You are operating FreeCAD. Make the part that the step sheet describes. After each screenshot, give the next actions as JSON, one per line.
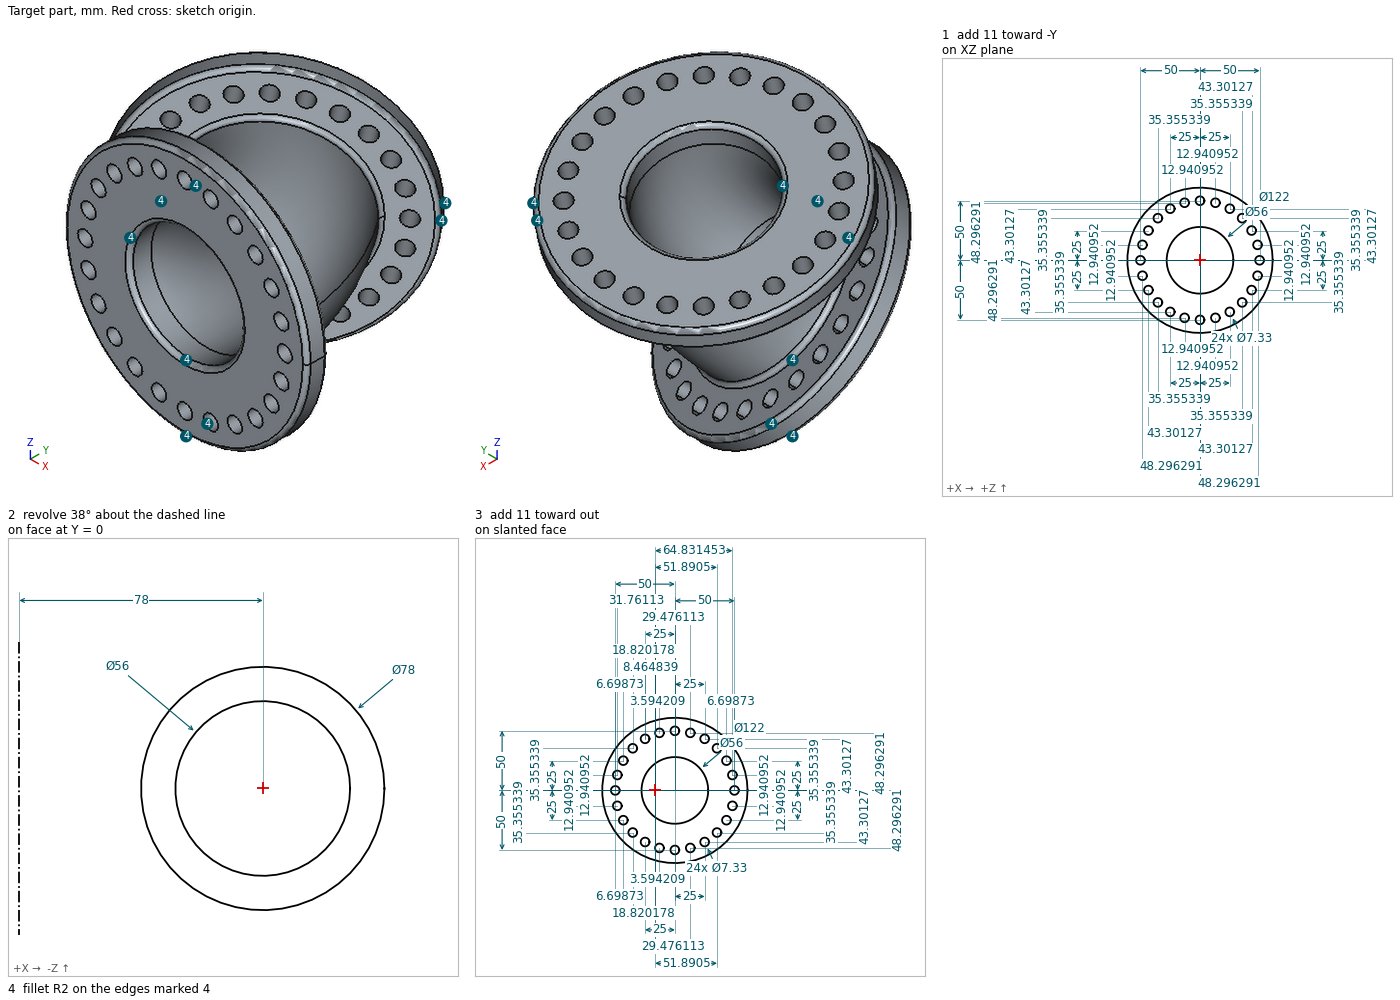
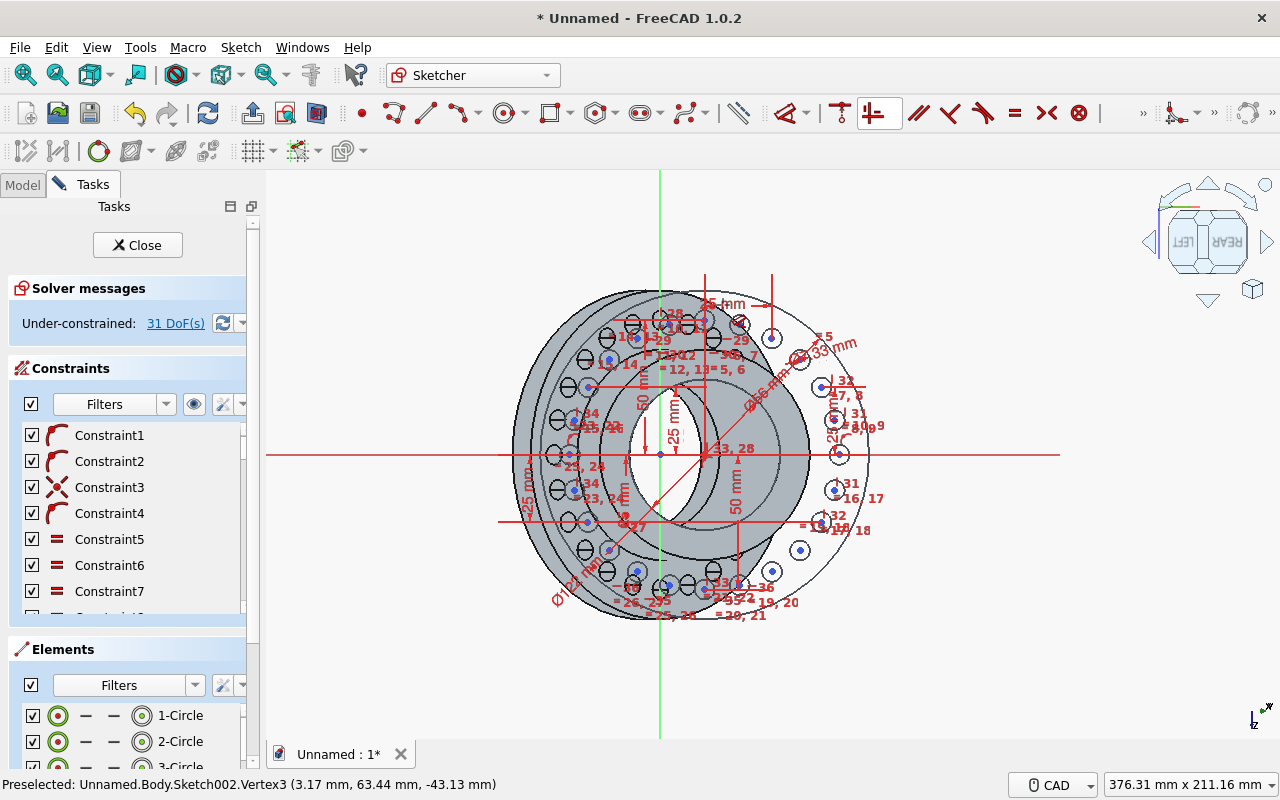
{"action": "left_click", "coordinate": [705, 455]}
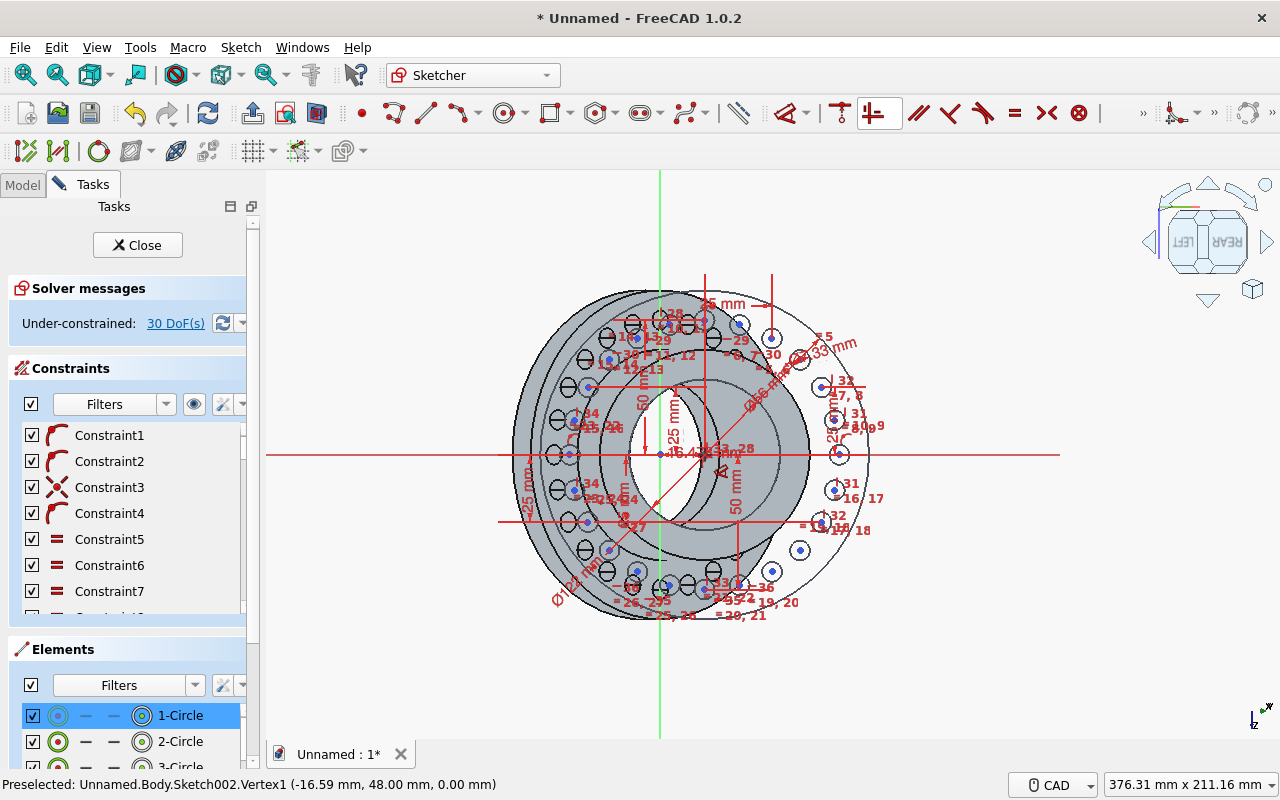
{"action": "left_click", "coordinate": [840, 455]}
{"action": "left_click", "coordinate": [772, 513]}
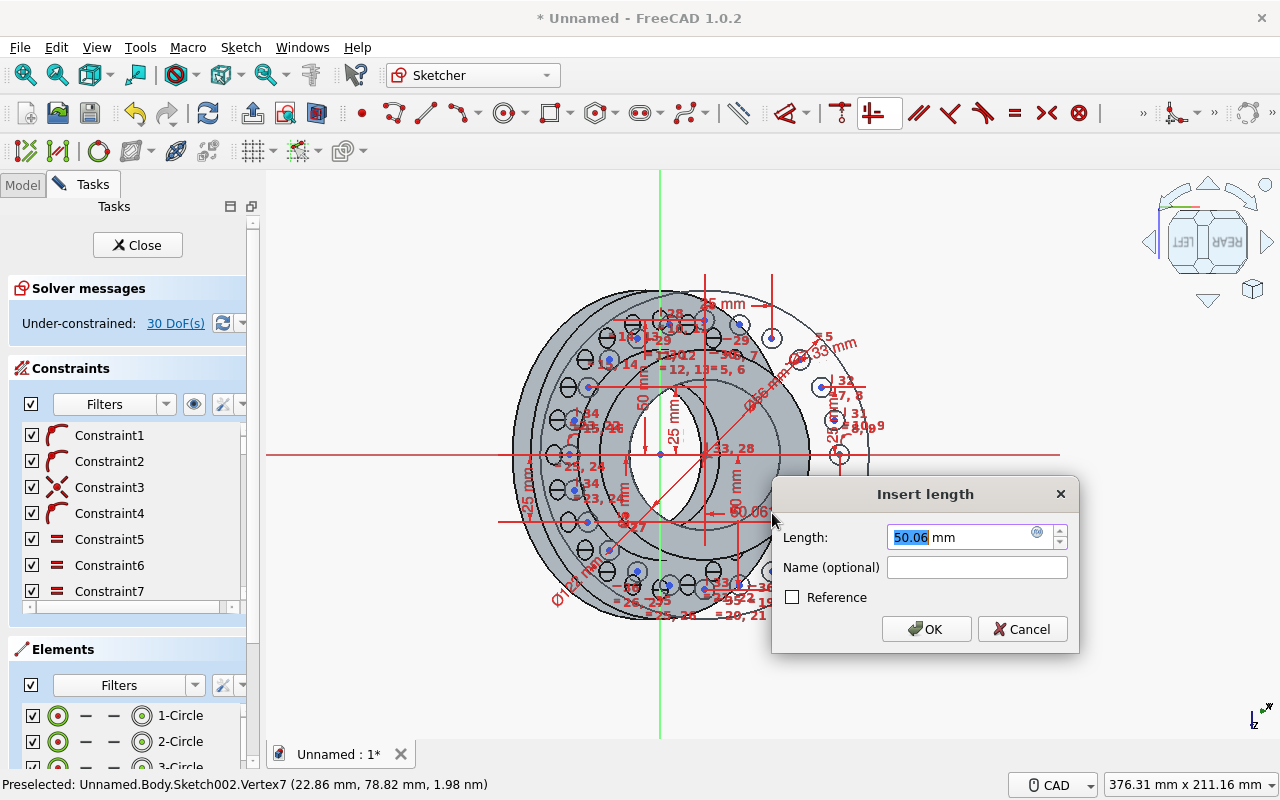
{"action": "type", "text": "50"}
{"action": "key", "text": "Return"}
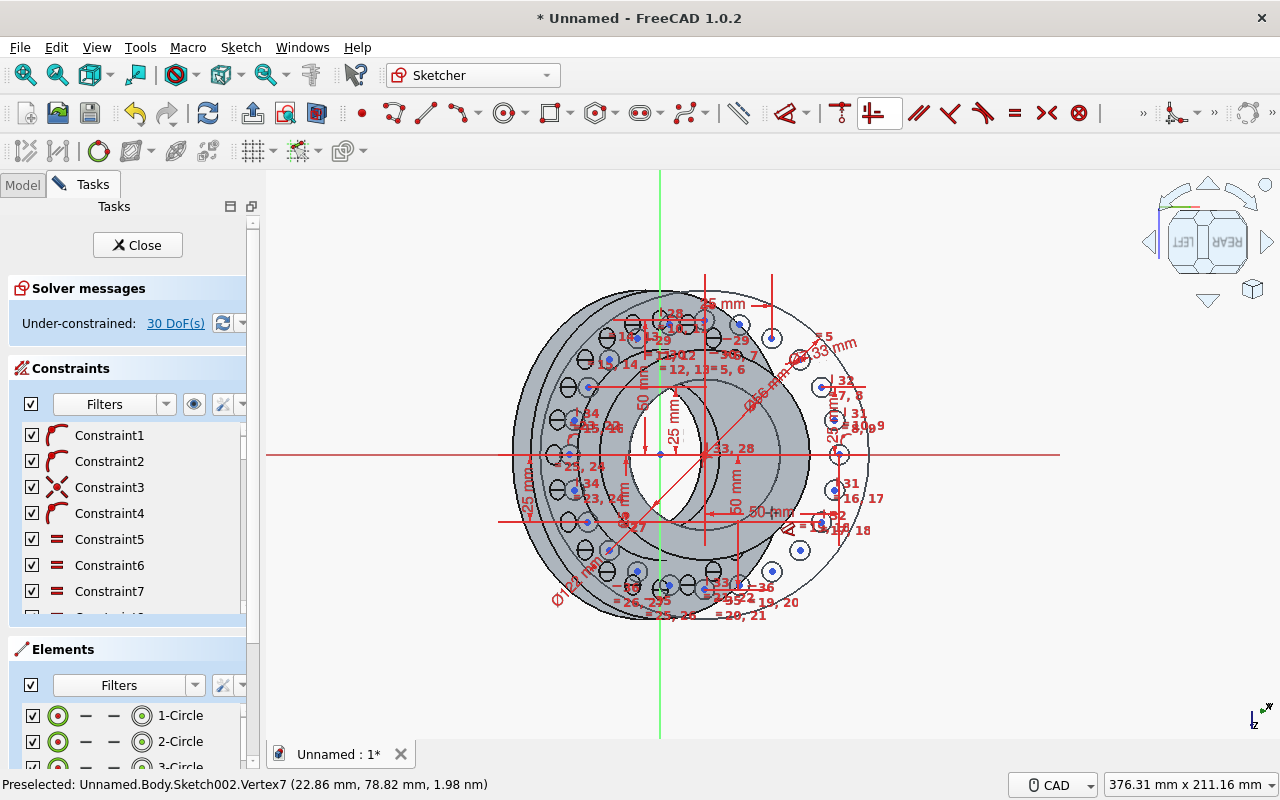
{"action": "left_click", "coordinate": [705, 320]}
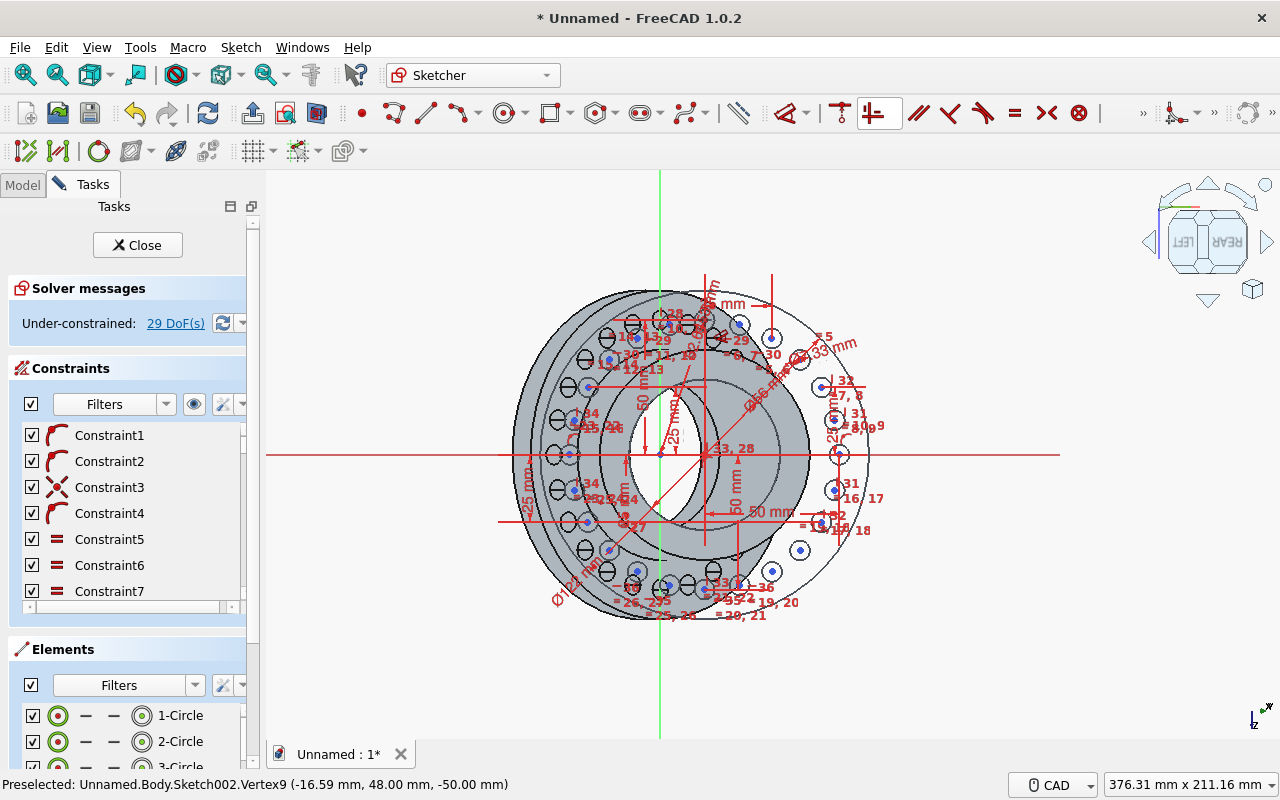
{"action": "left_click", "coordinate": [638, 339]}
{"action": "left_click", "coordinate": [687, 262]}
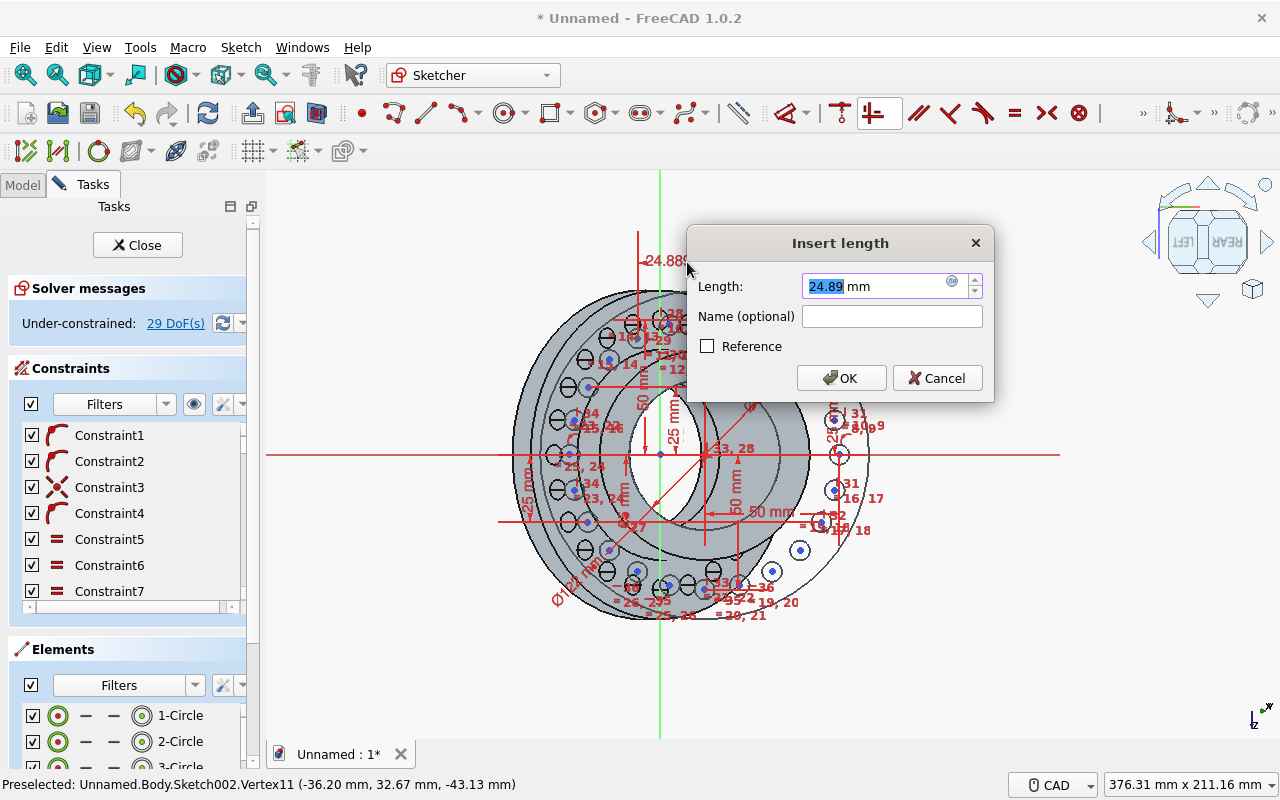
{"action": "type", "text": "25"}
{"action": "key", "text": "Return"}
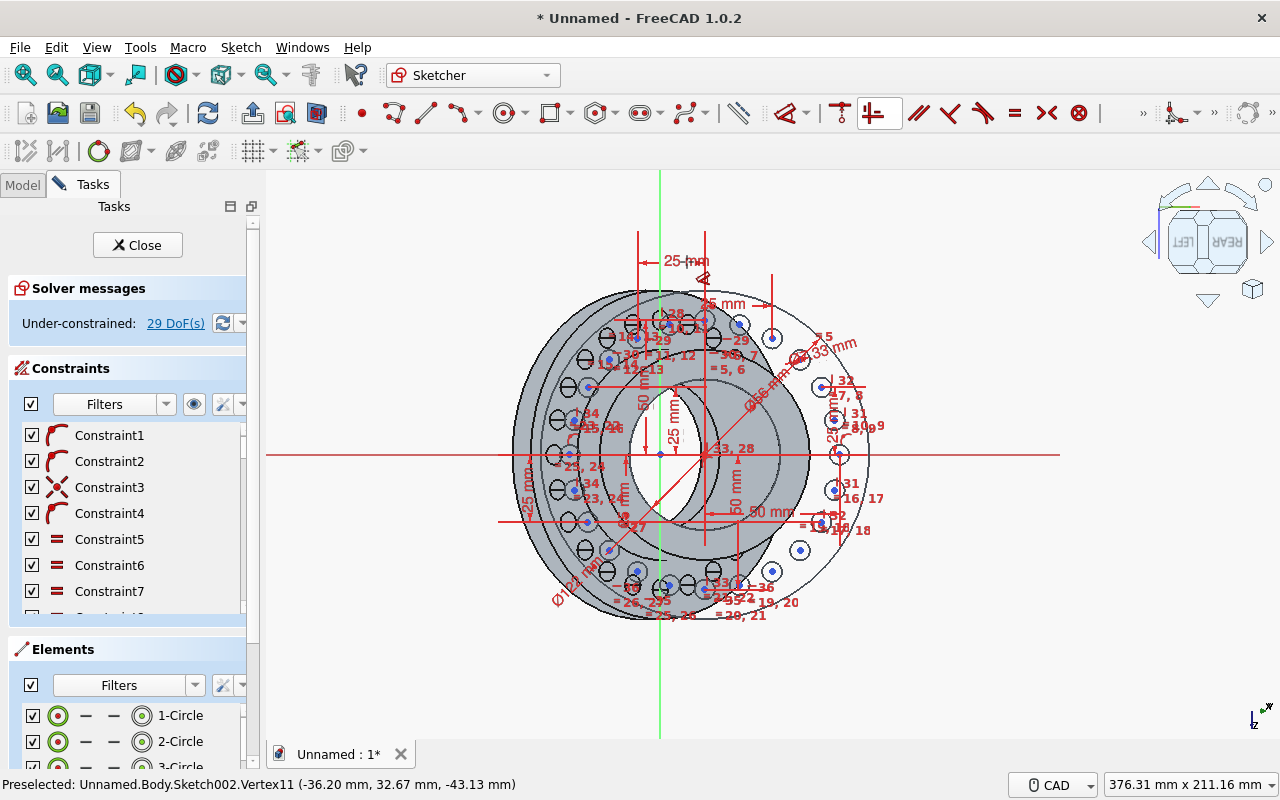
{"action": "left_click", "coordinate": [705, 455]}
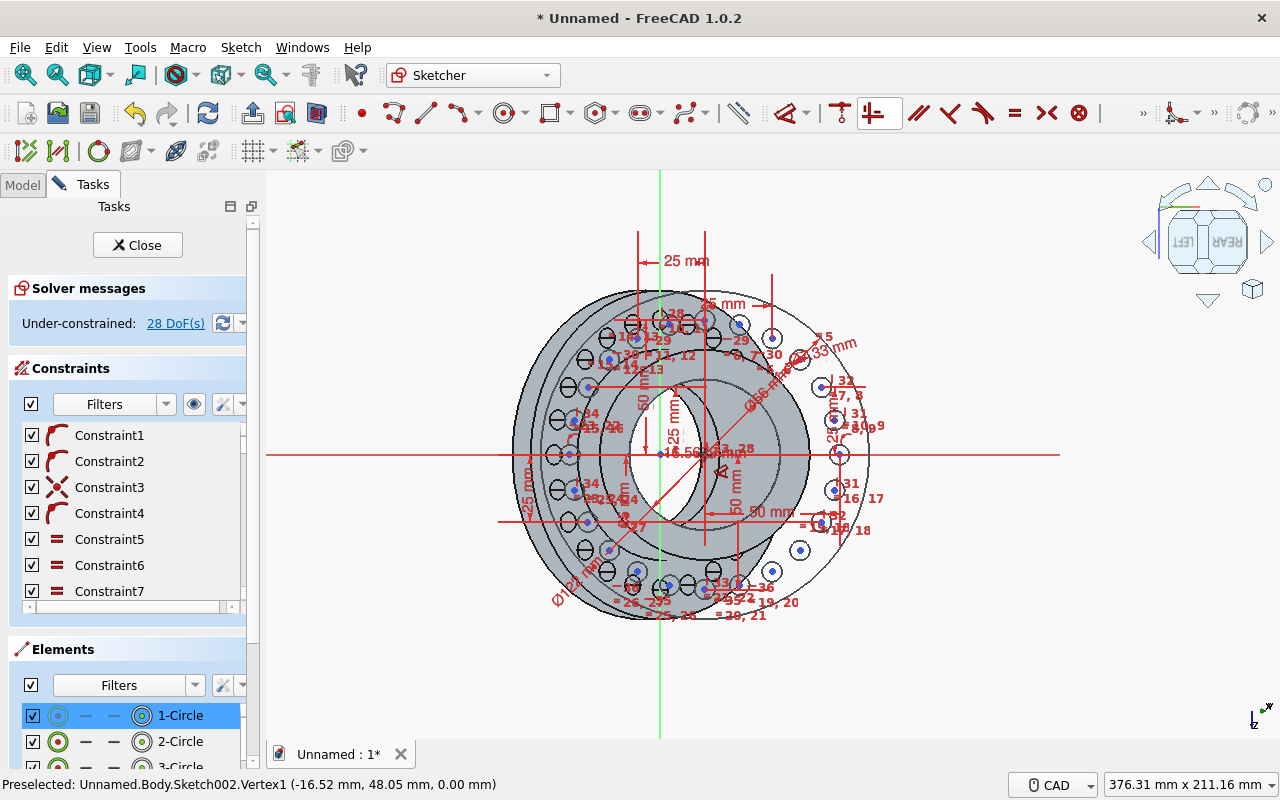
{"action": "left_click", "coordinate": [772, 572]}
{"action": "left_click", "coordinate": [754, 421]}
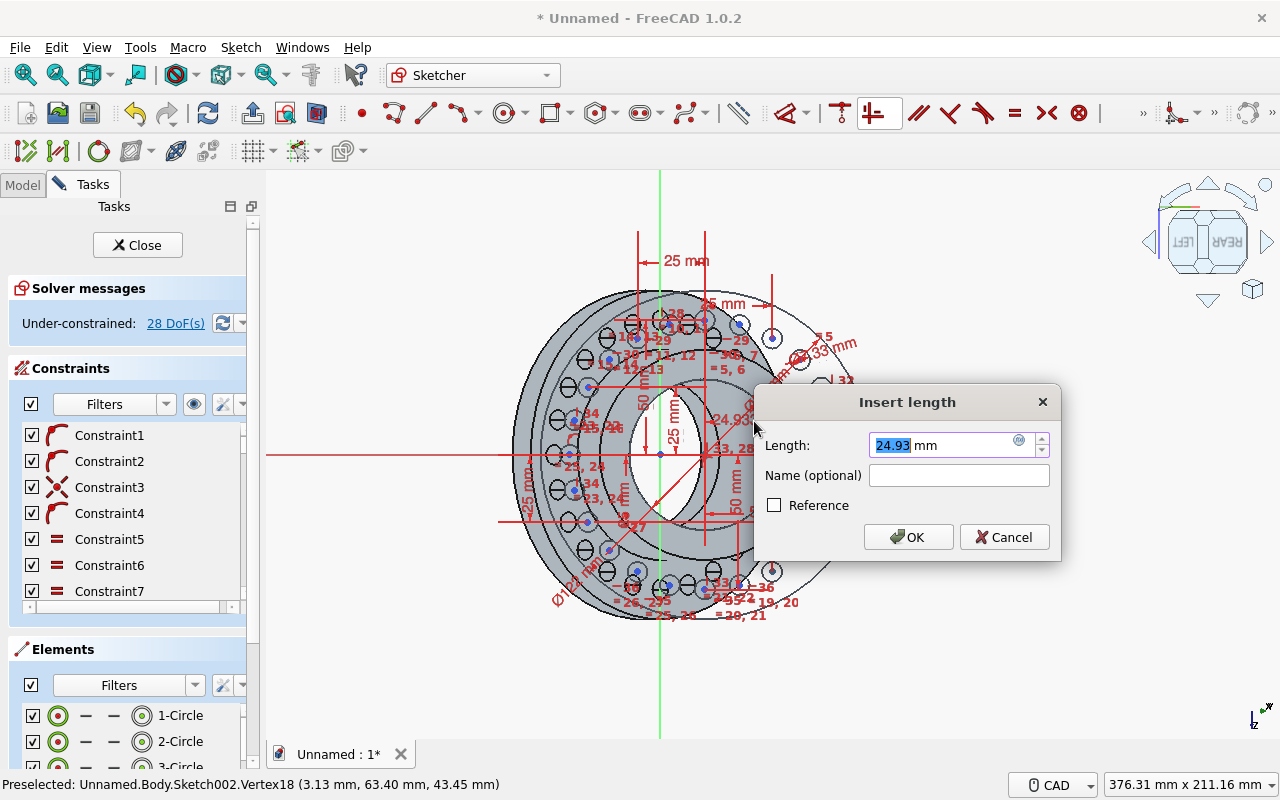
{"action": "type", "text": "25"}
{"action": "key", "text": "Return"}